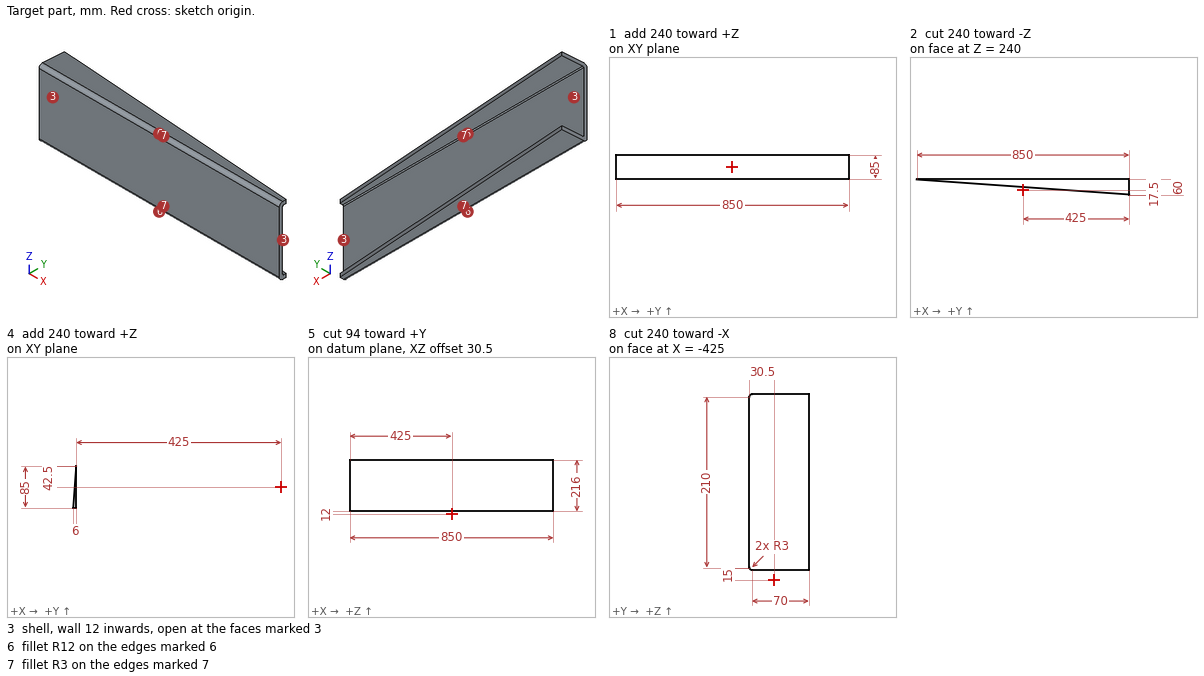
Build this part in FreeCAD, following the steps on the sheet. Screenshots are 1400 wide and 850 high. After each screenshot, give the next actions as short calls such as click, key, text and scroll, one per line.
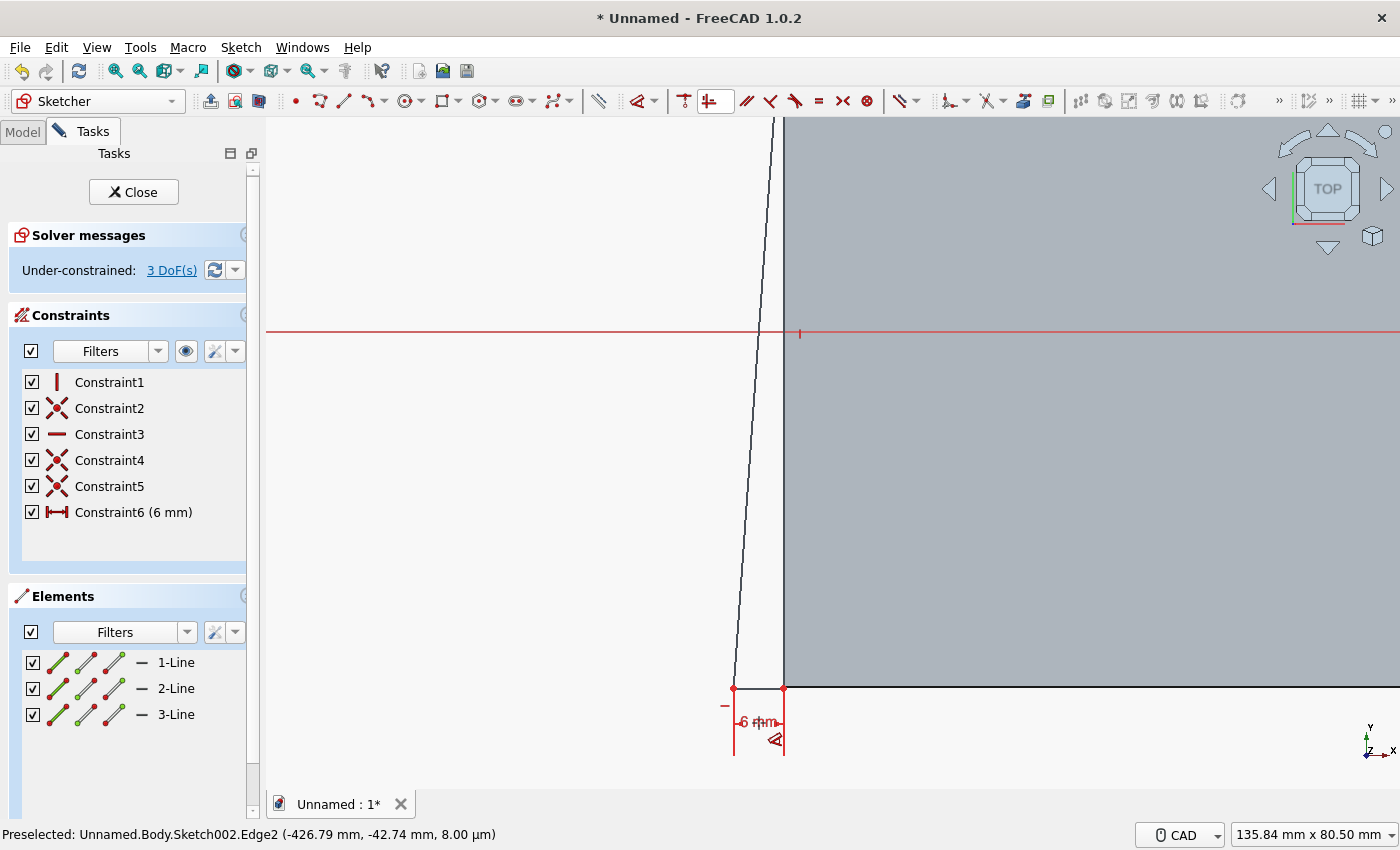
click(784, 192)
click(818, 417)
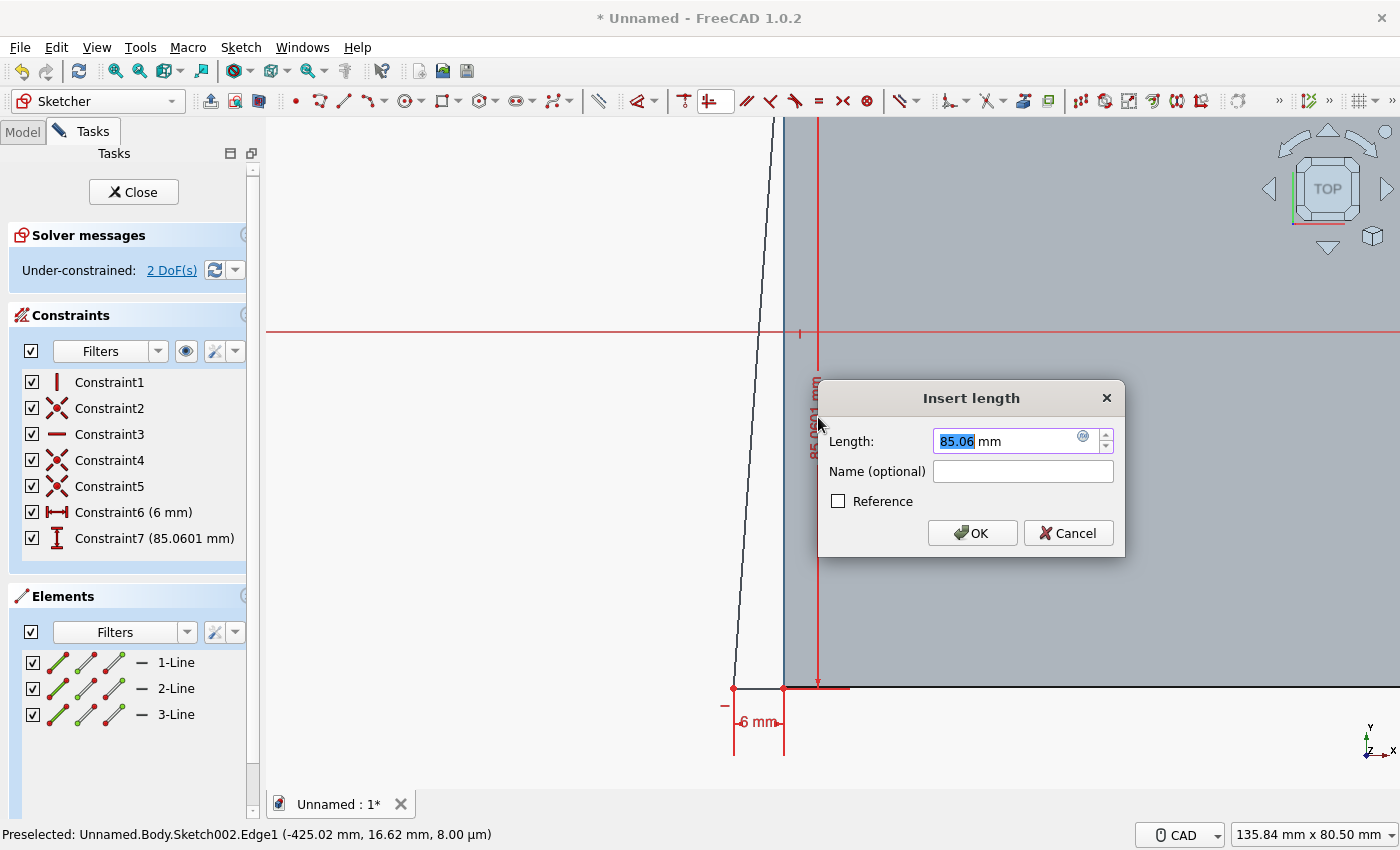
text(85)
key(Return)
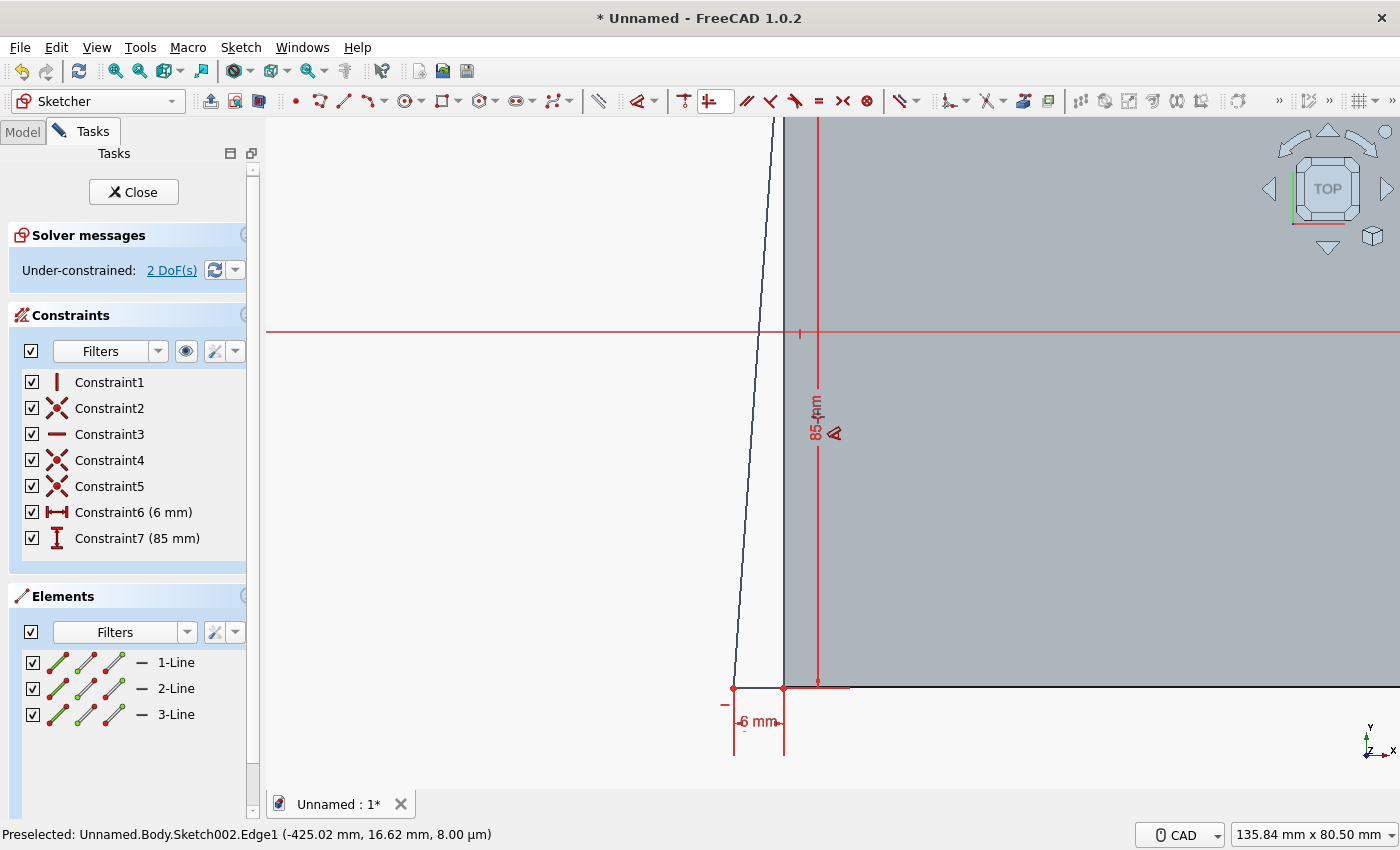
scroll(776, 700, down, 2)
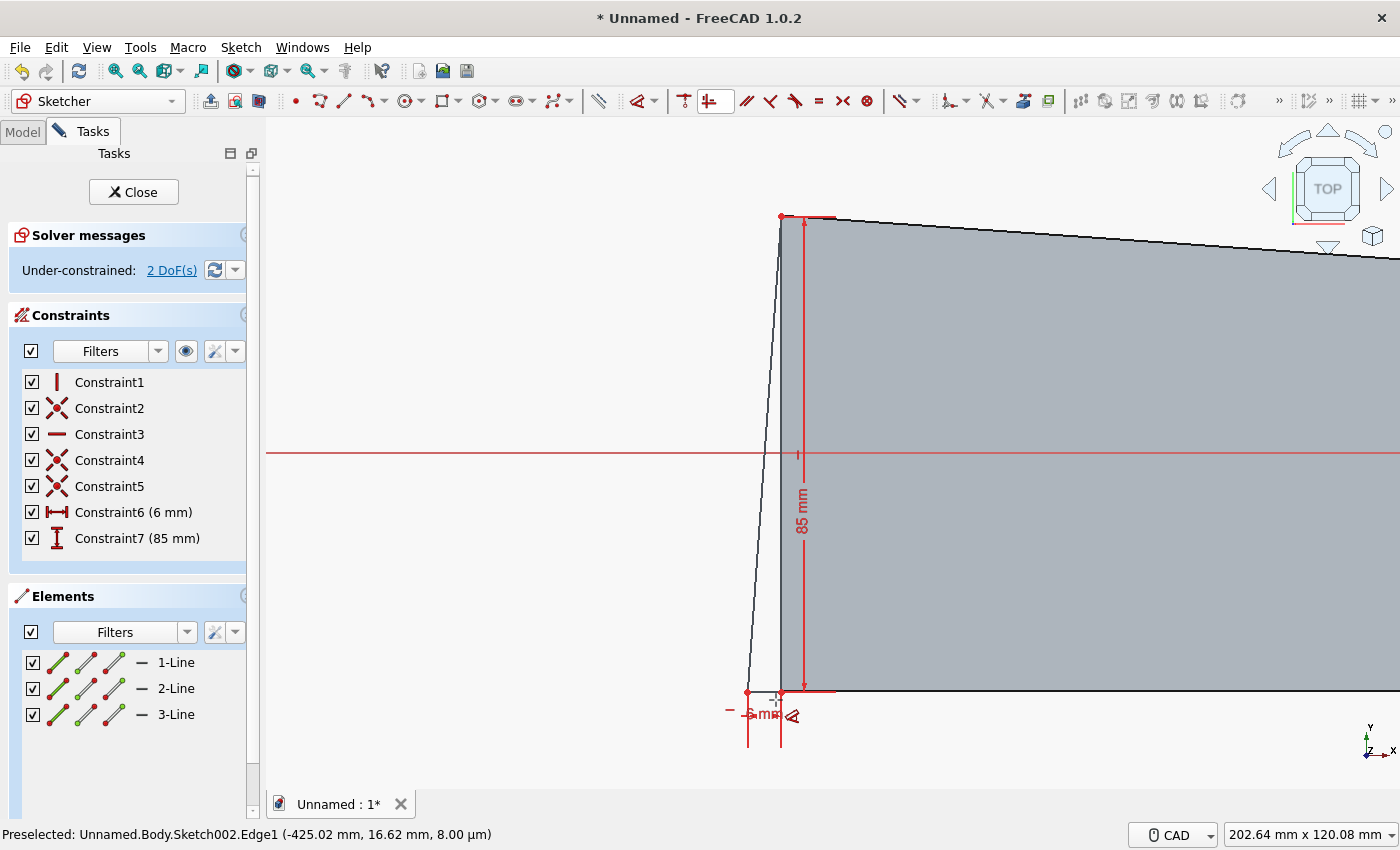
click(781, 217)
click(1008, 183)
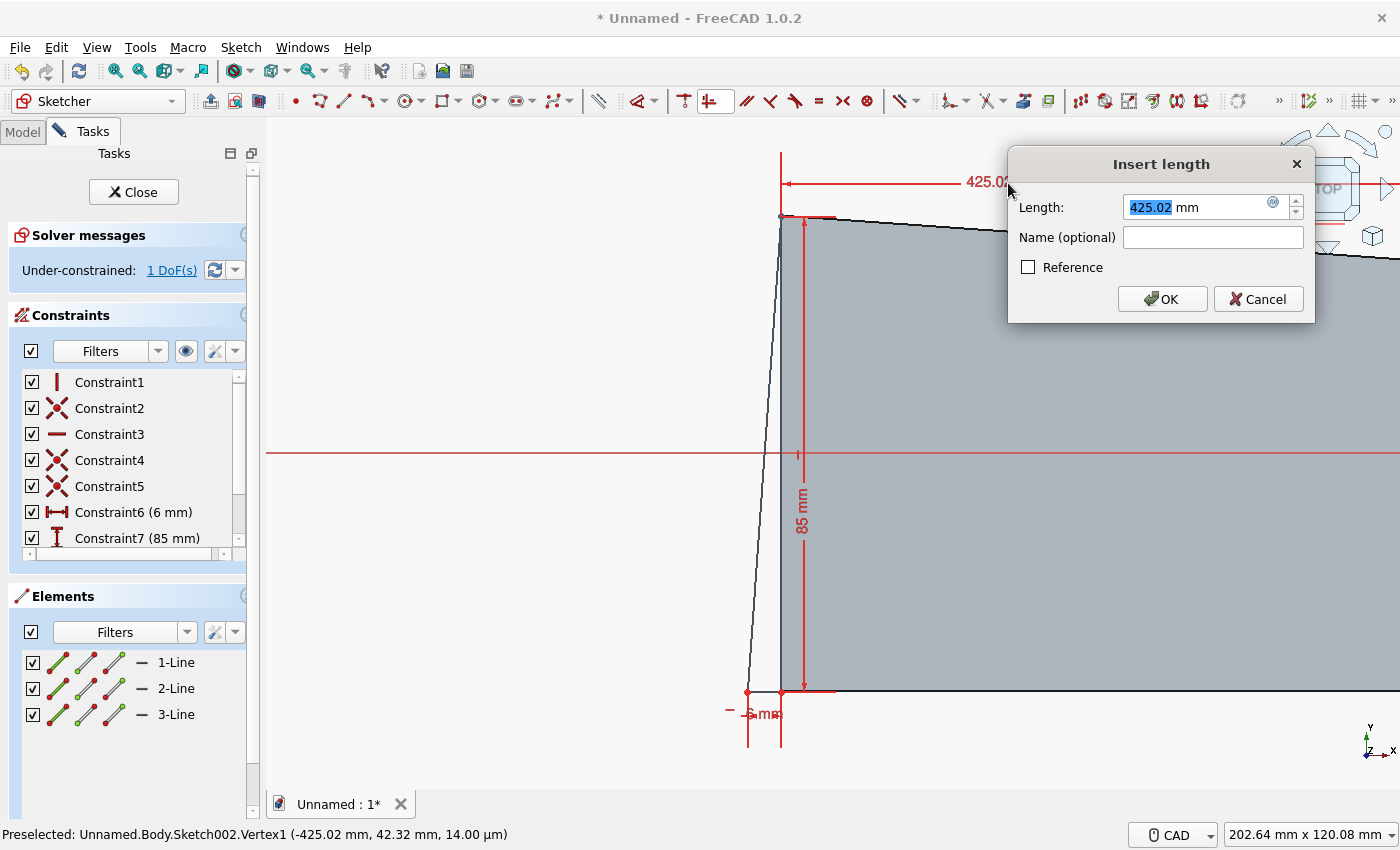
text(425)
key(Return)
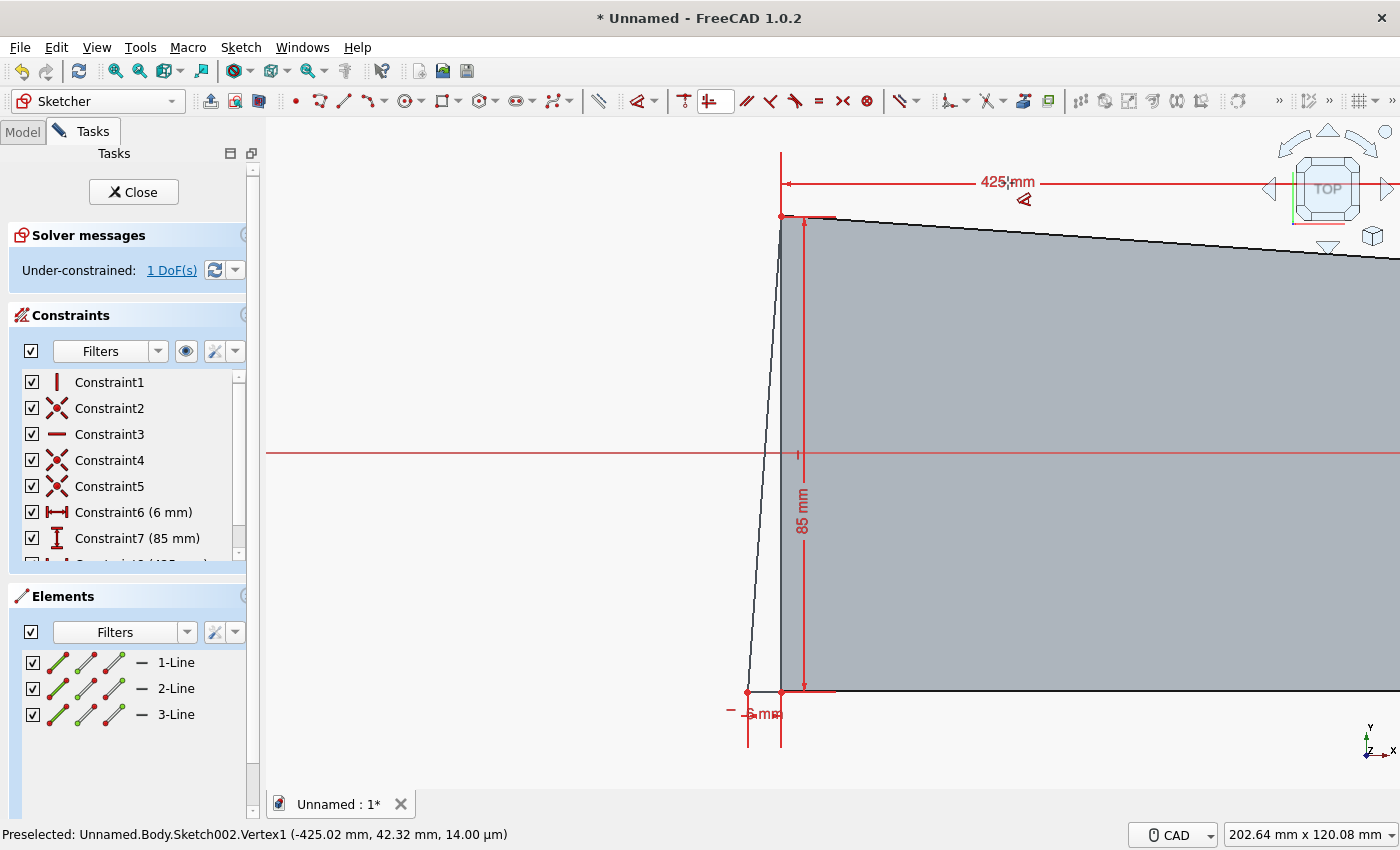
click(781, 217)
click(747, 335)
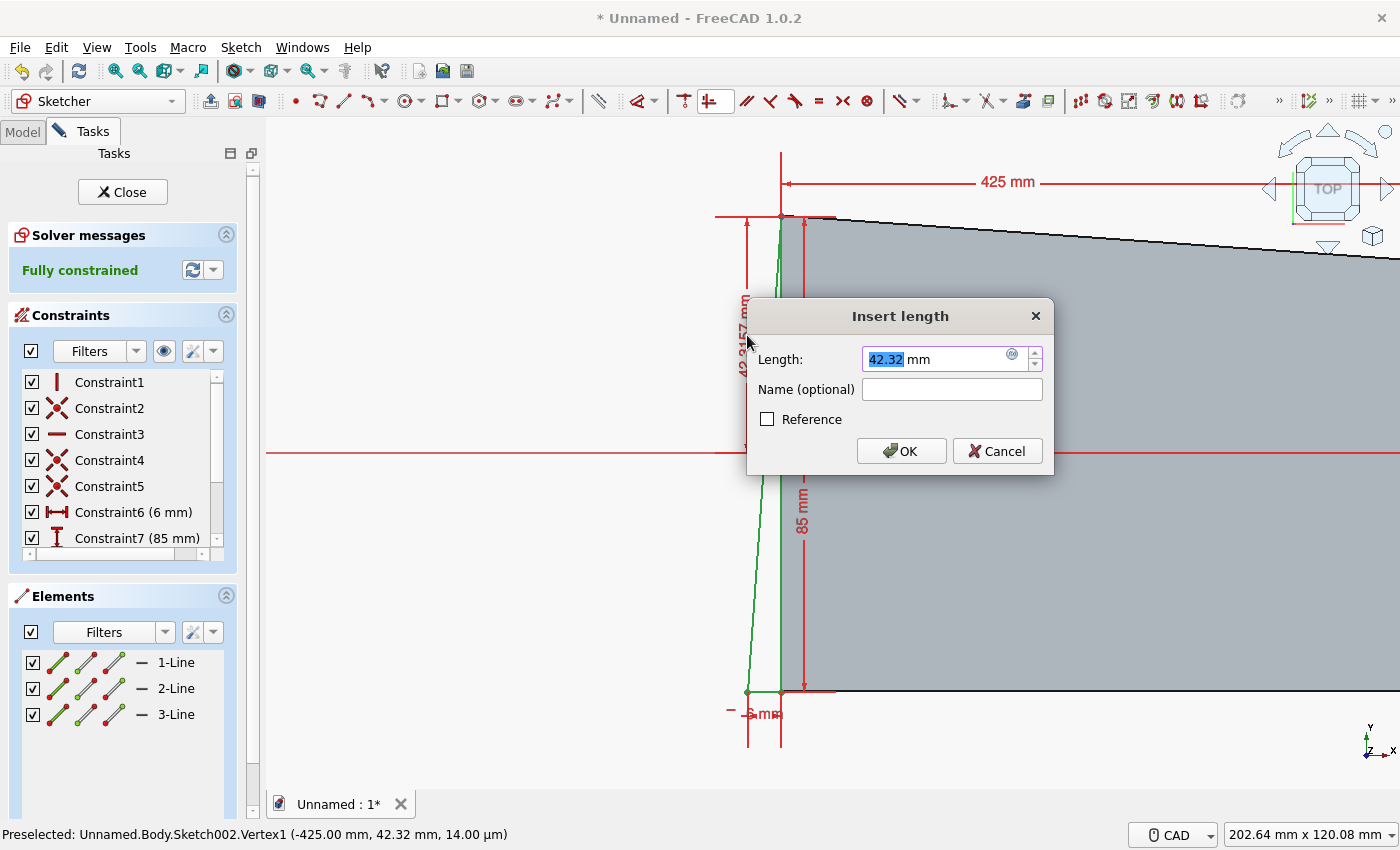
text(42.5)
key(Return)
key(Escape)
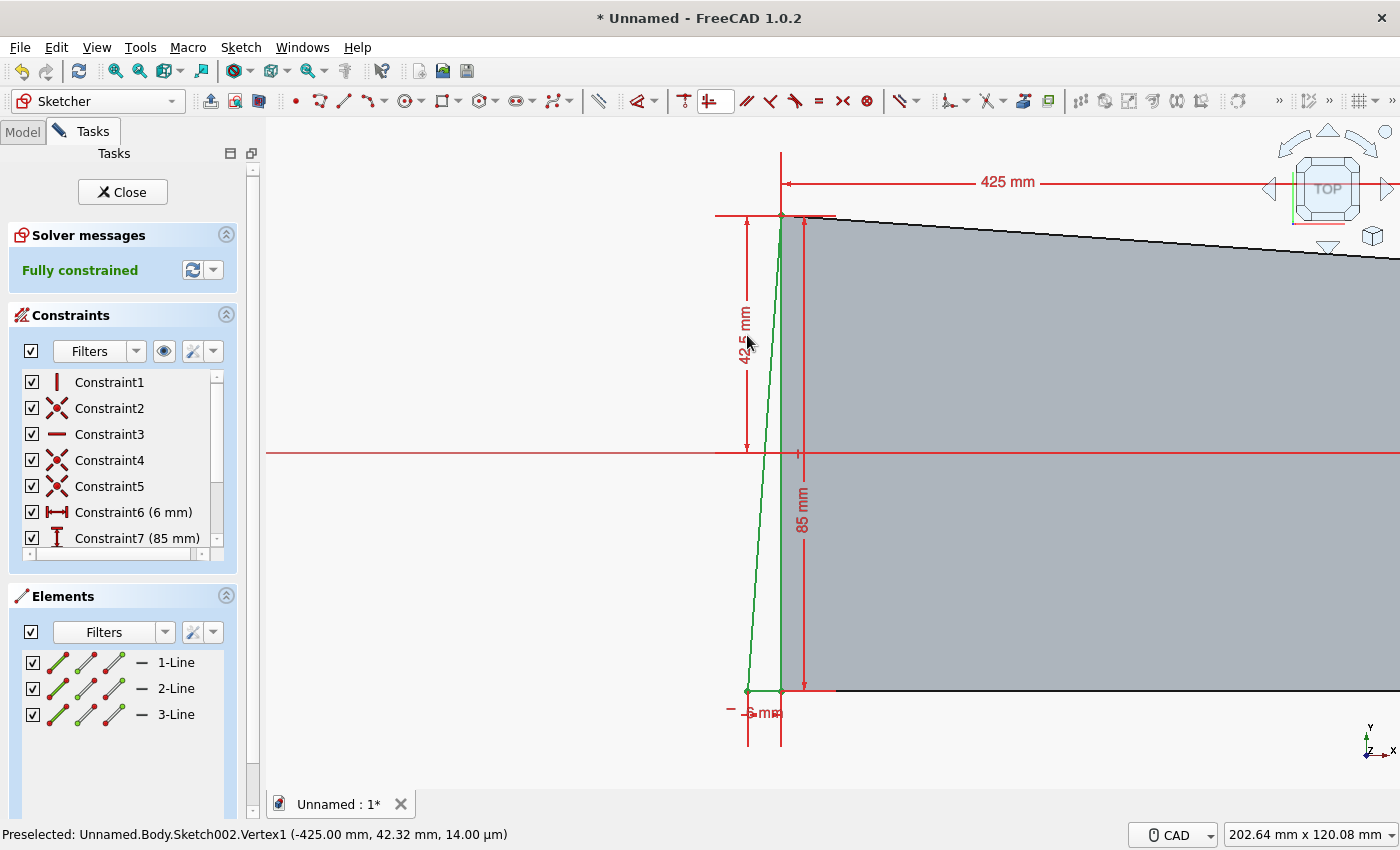
click(123, 192)